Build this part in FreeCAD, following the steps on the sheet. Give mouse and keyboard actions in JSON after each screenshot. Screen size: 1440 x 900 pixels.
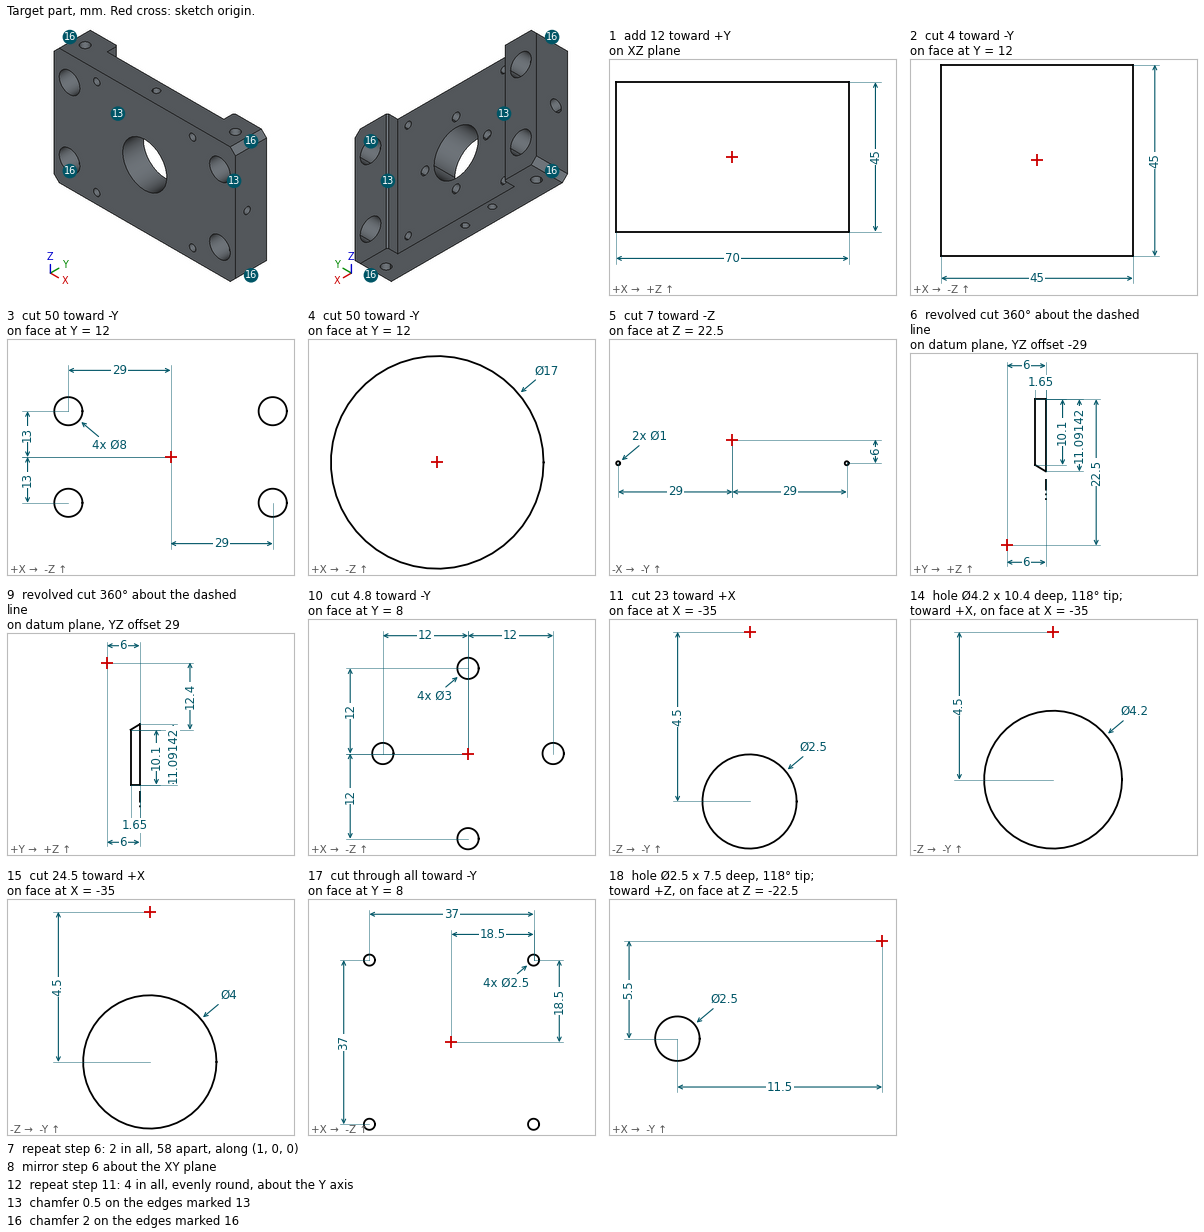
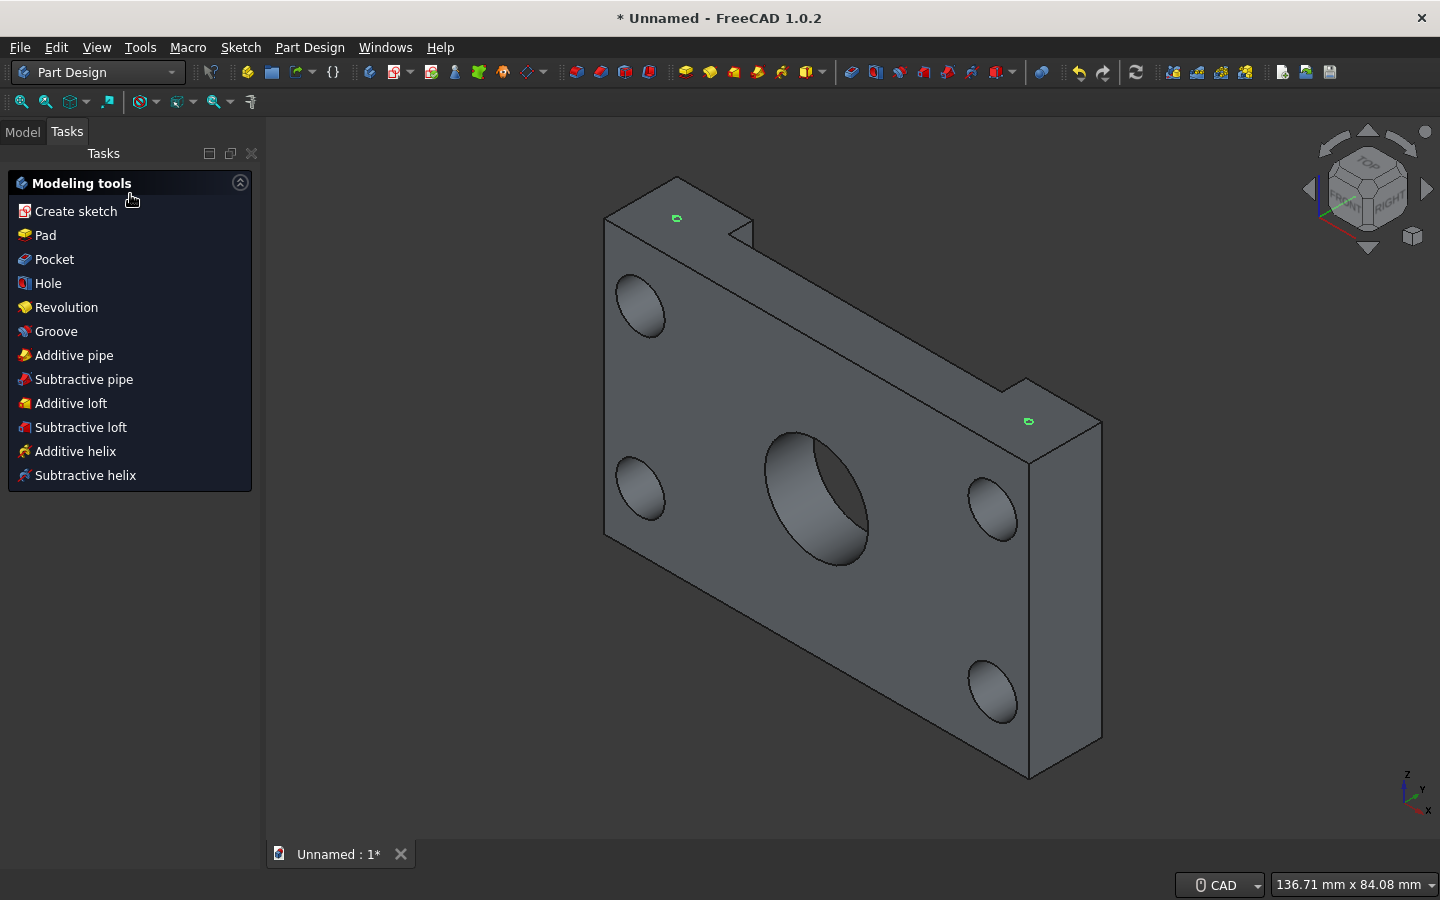
{"action": "left_click", "coordinate": [852, 72]}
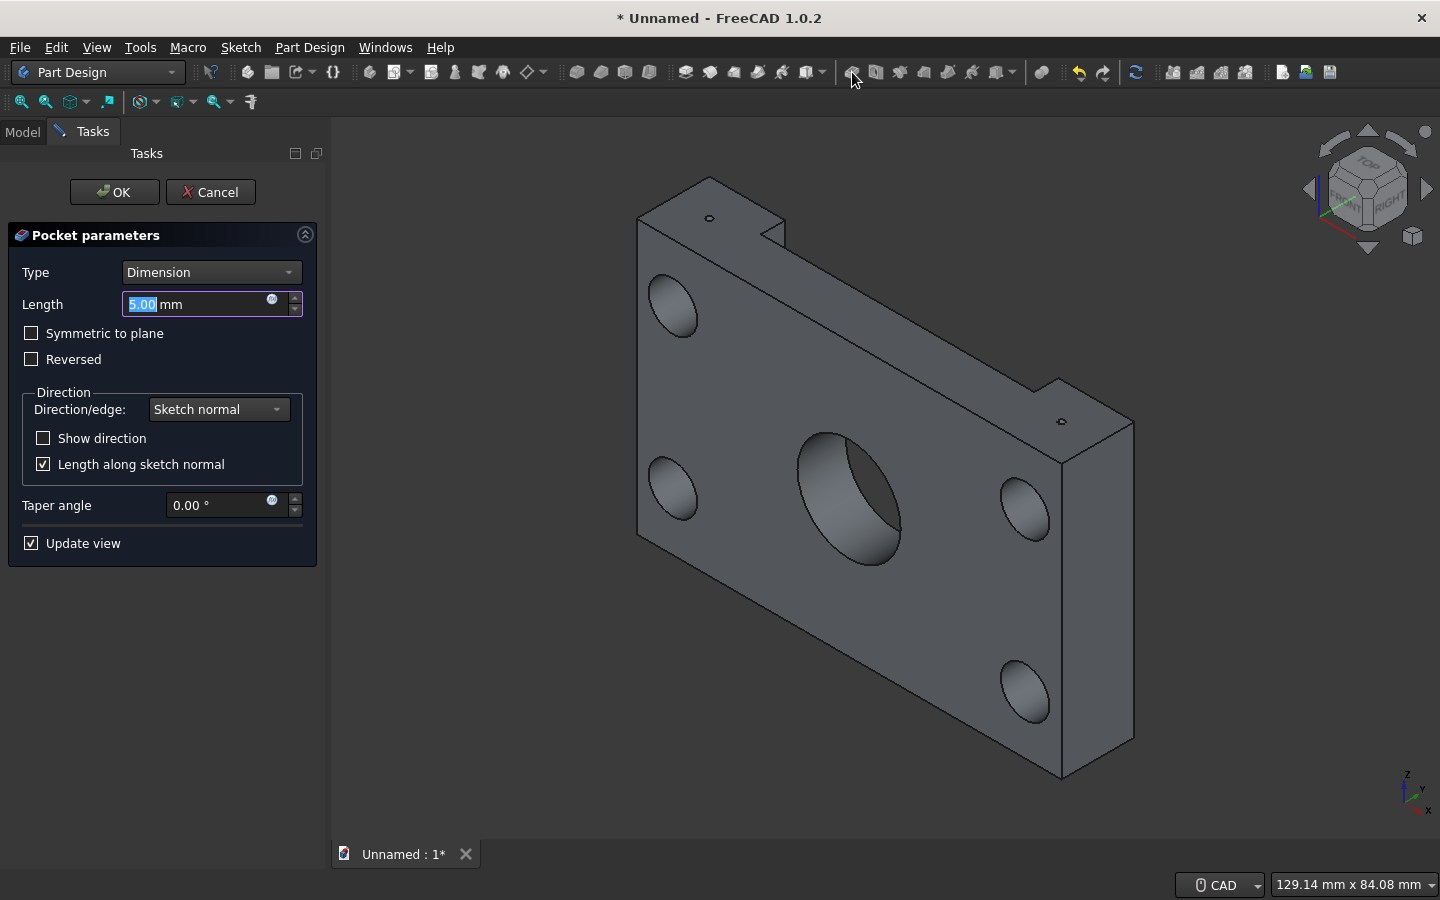
{"action": "type", "text": "7"}
{"action": "key", "text": "Tab"}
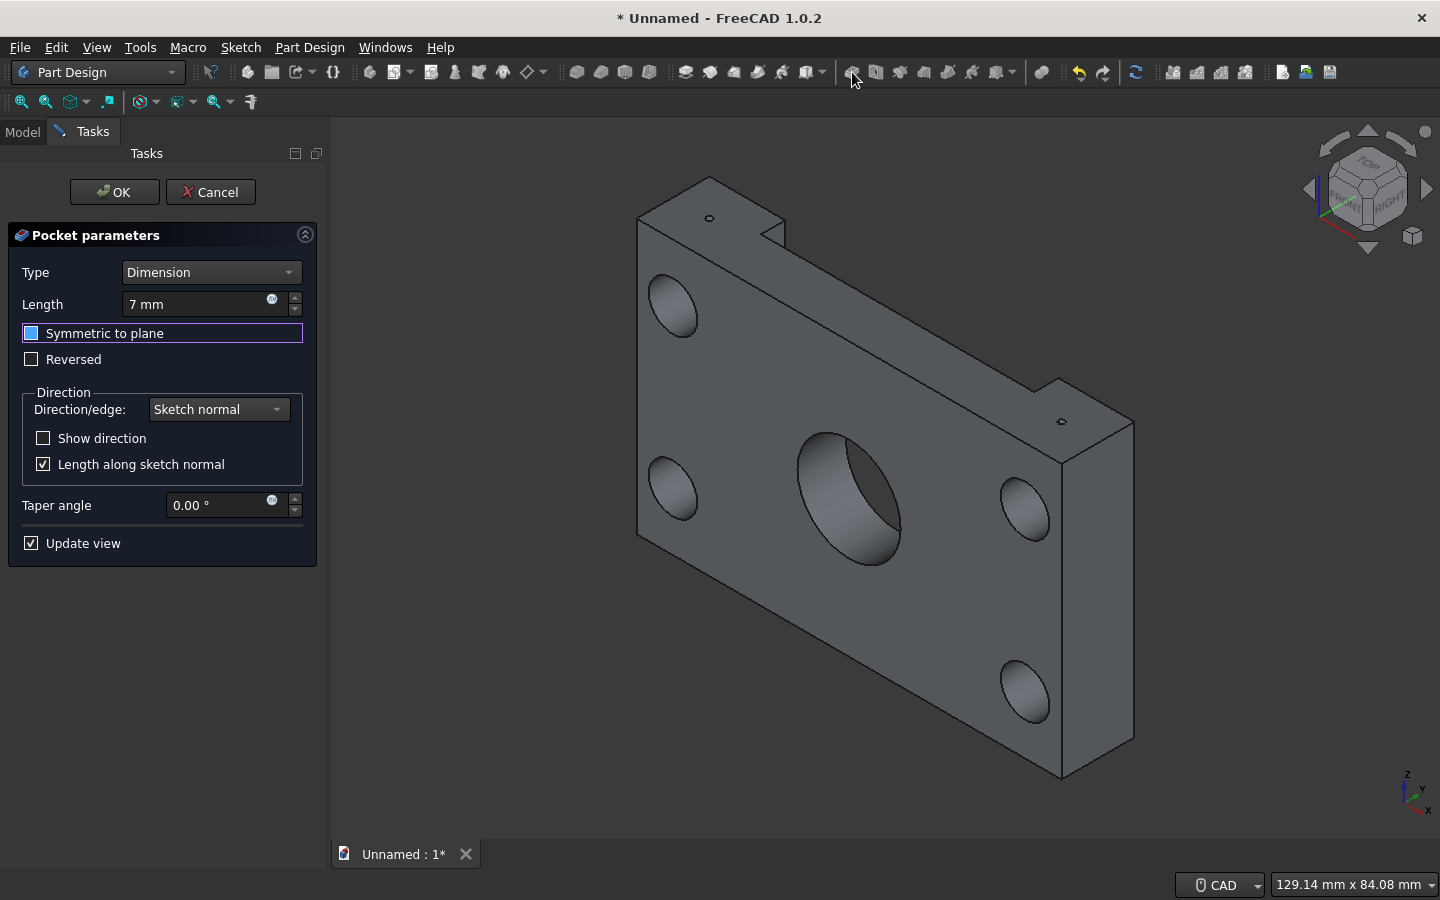
{"action": "left_click", "coordinate": [115, 192]}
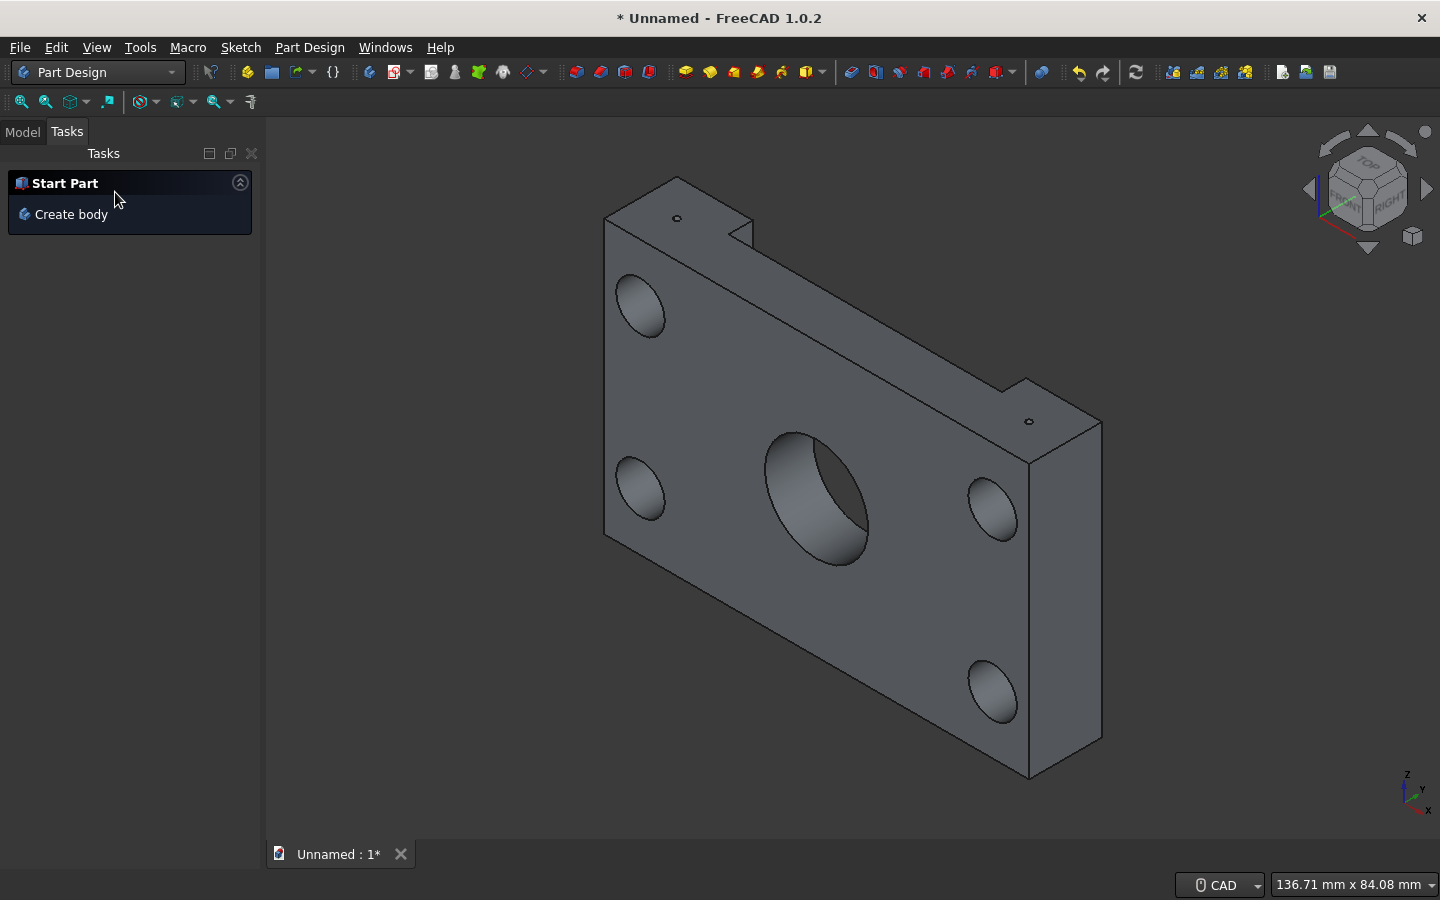
{"action": "left_click", "coordinate": [23, 131]}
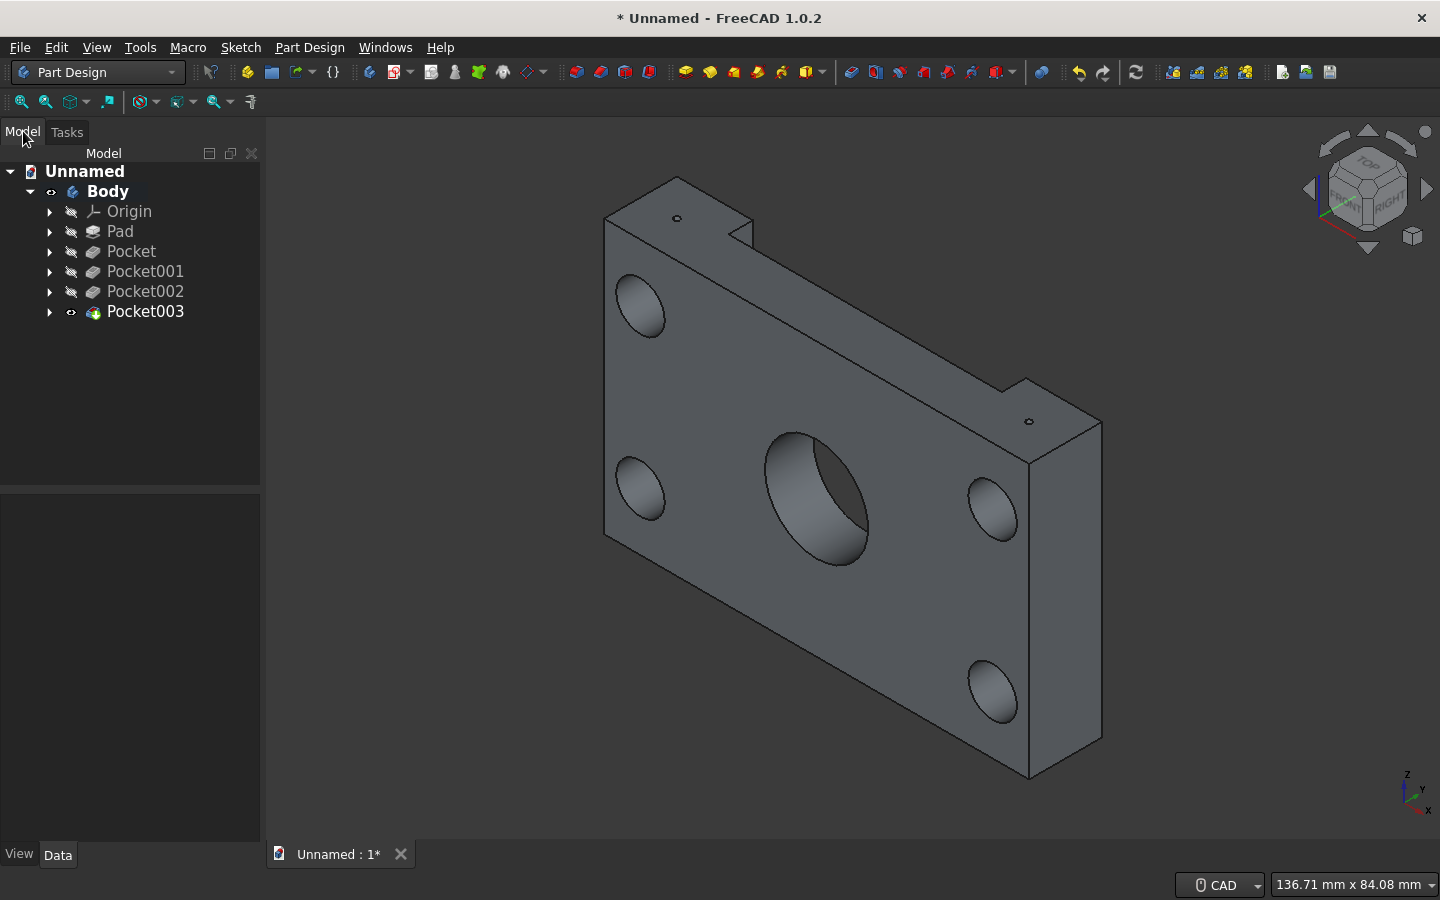
{"action": "left_click", "coordinate": [50, 212]}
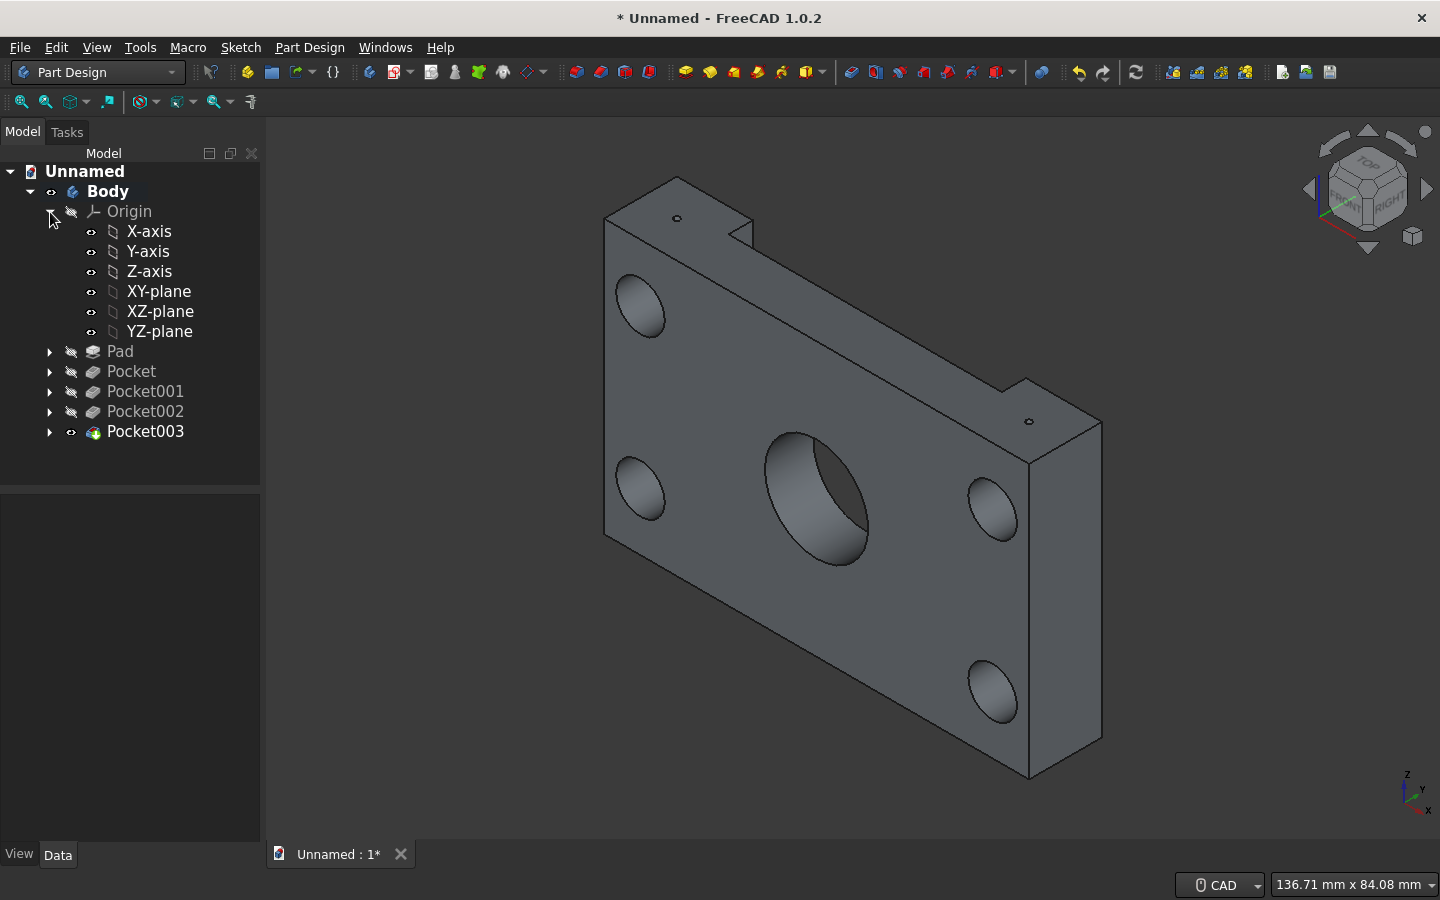
{"action": "left_click", "coordinate": [136, 332]}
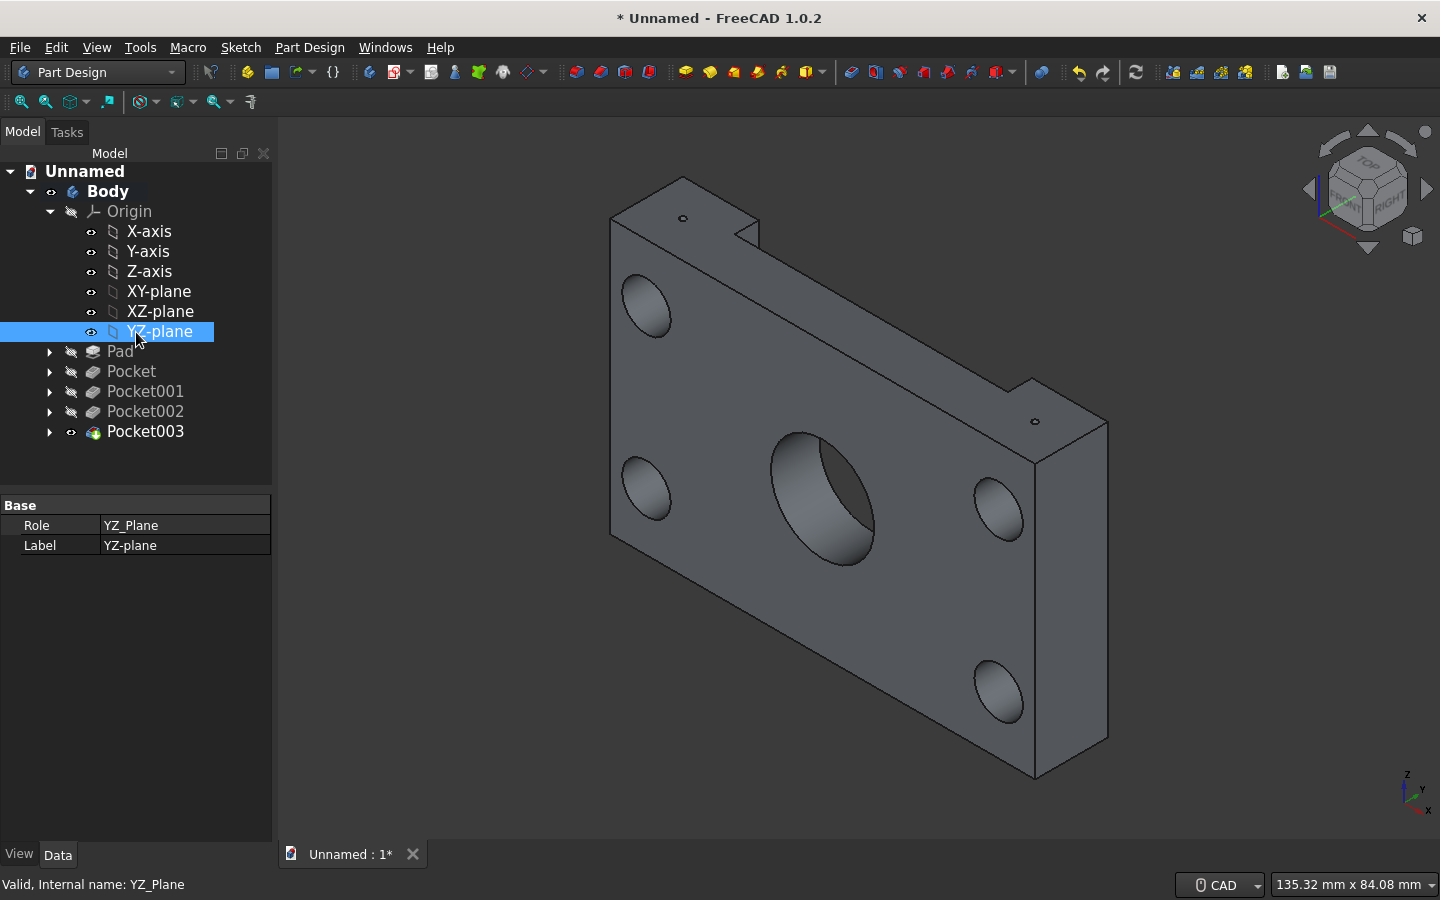
{"action": "left_click", "coordinate": [528, 72]}